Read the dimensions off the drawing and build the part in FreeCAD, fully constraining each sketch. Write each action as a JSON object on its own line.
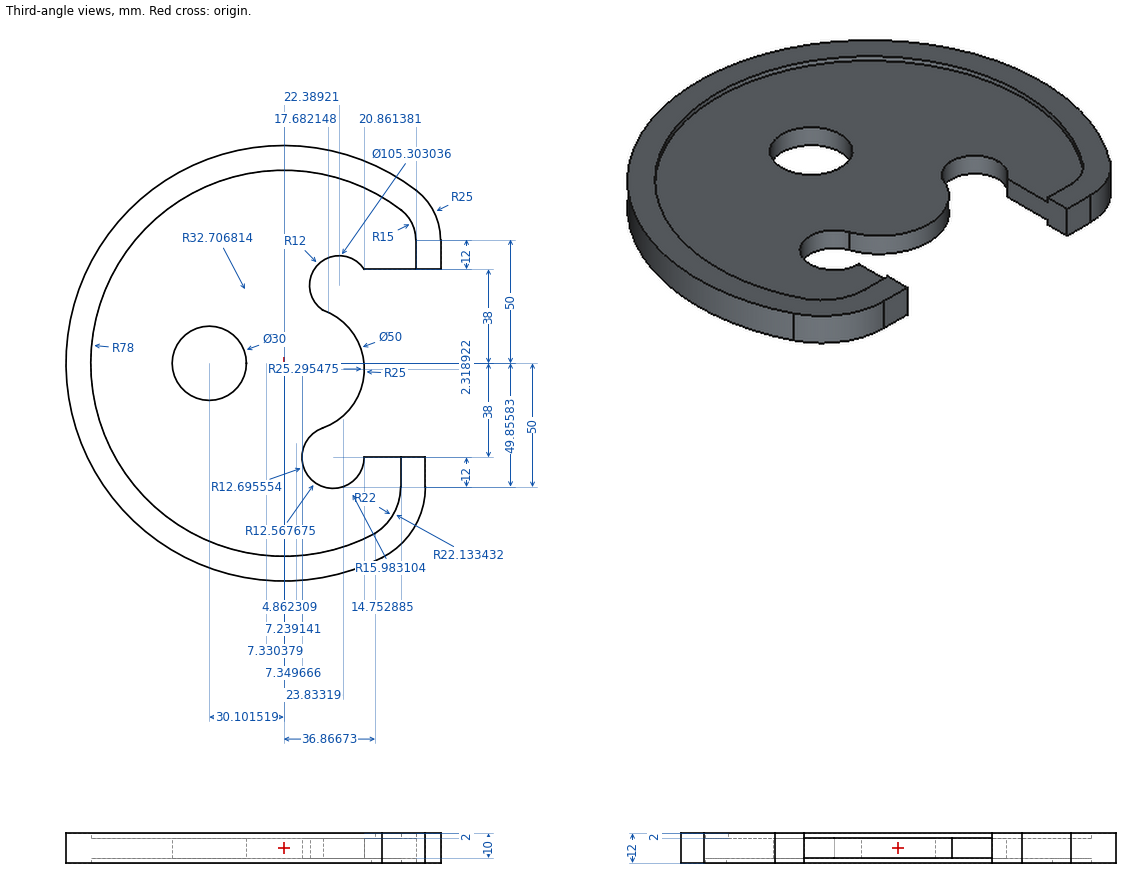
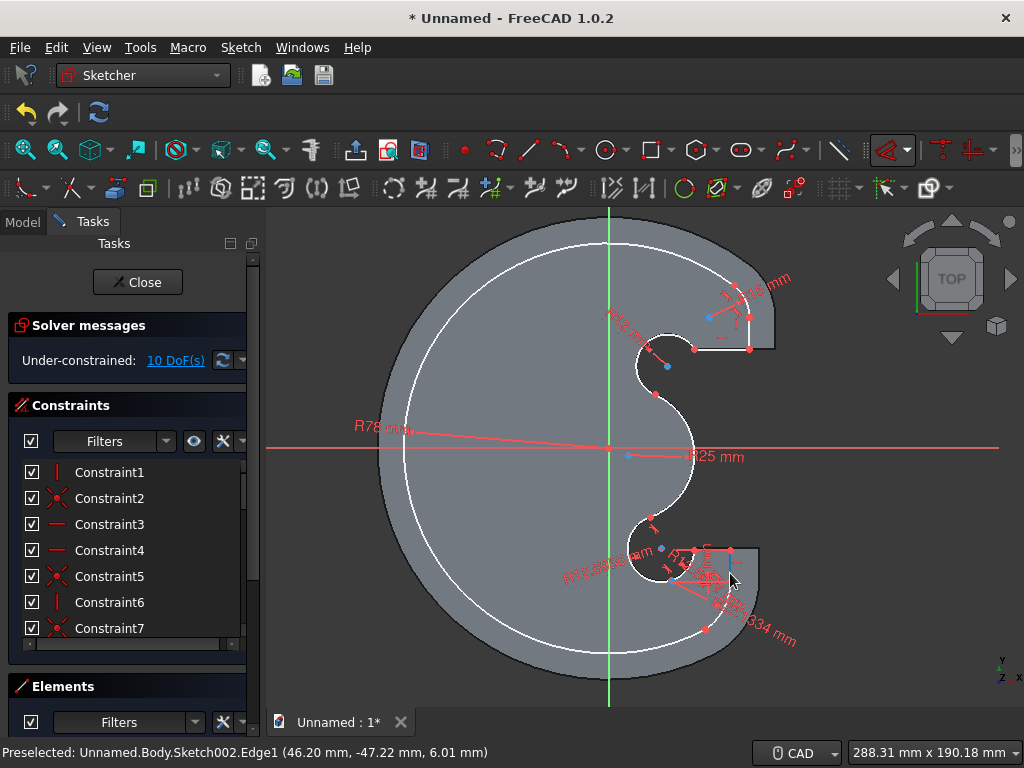
{"action": "scroll", "coordinate": [749, 340], "scroll_direction": "up", "scroll_amount": 2}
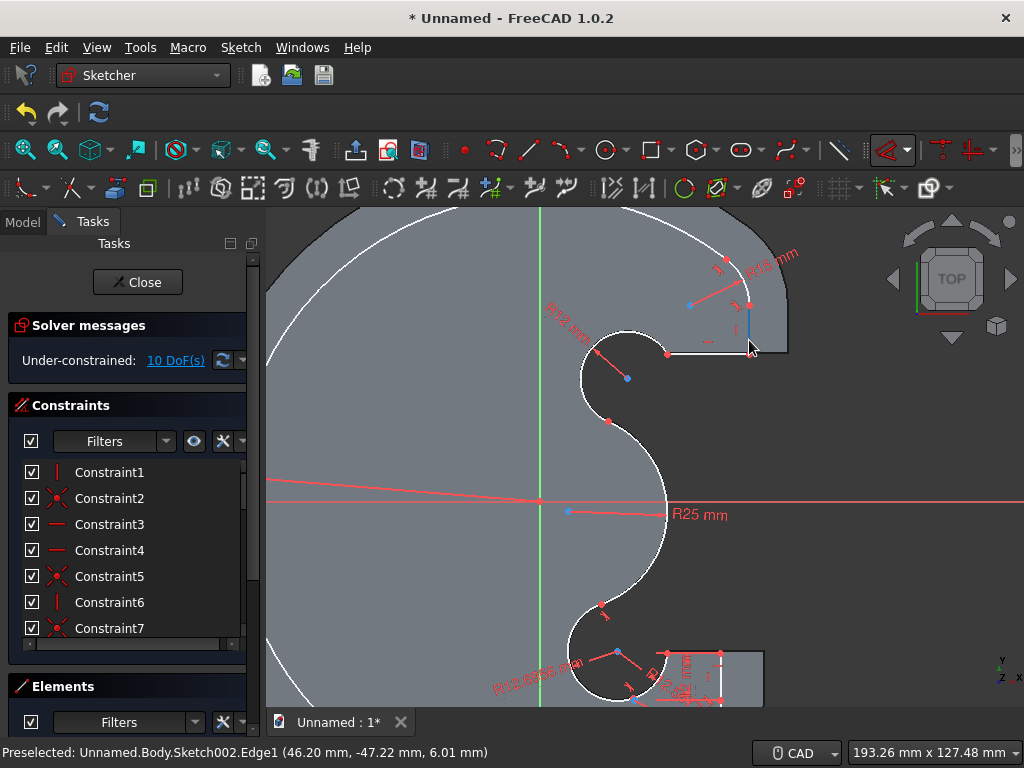
{"action": "left_click", "coordinate": [749, 340]}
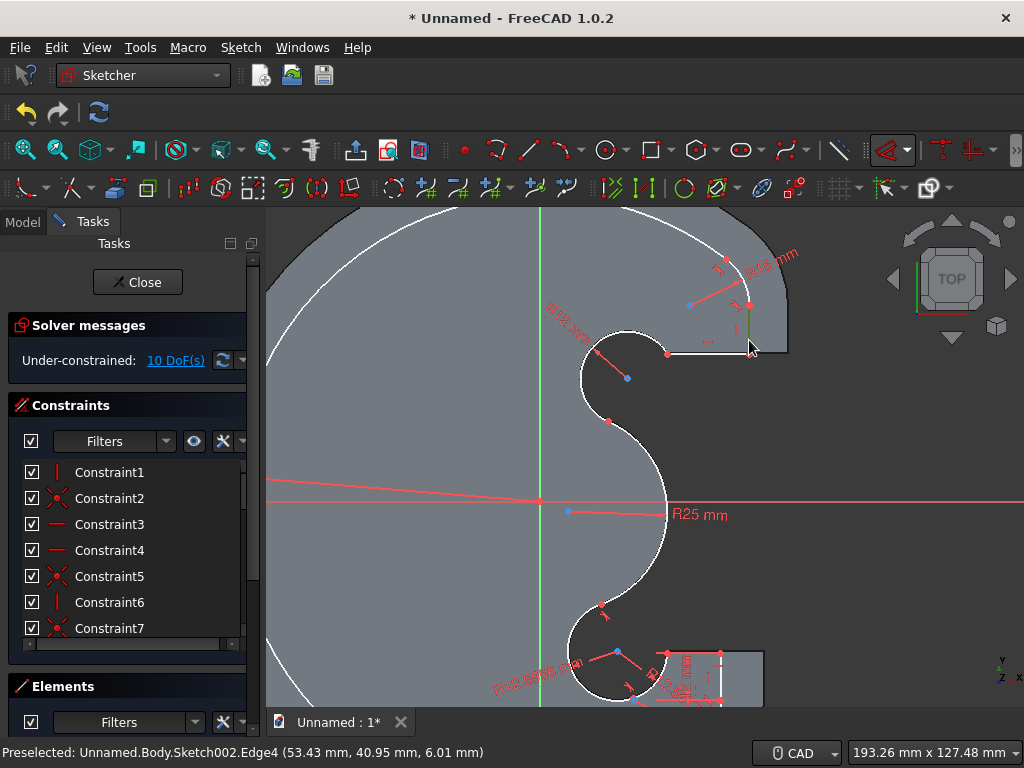
{"action": "key", "text": "i"}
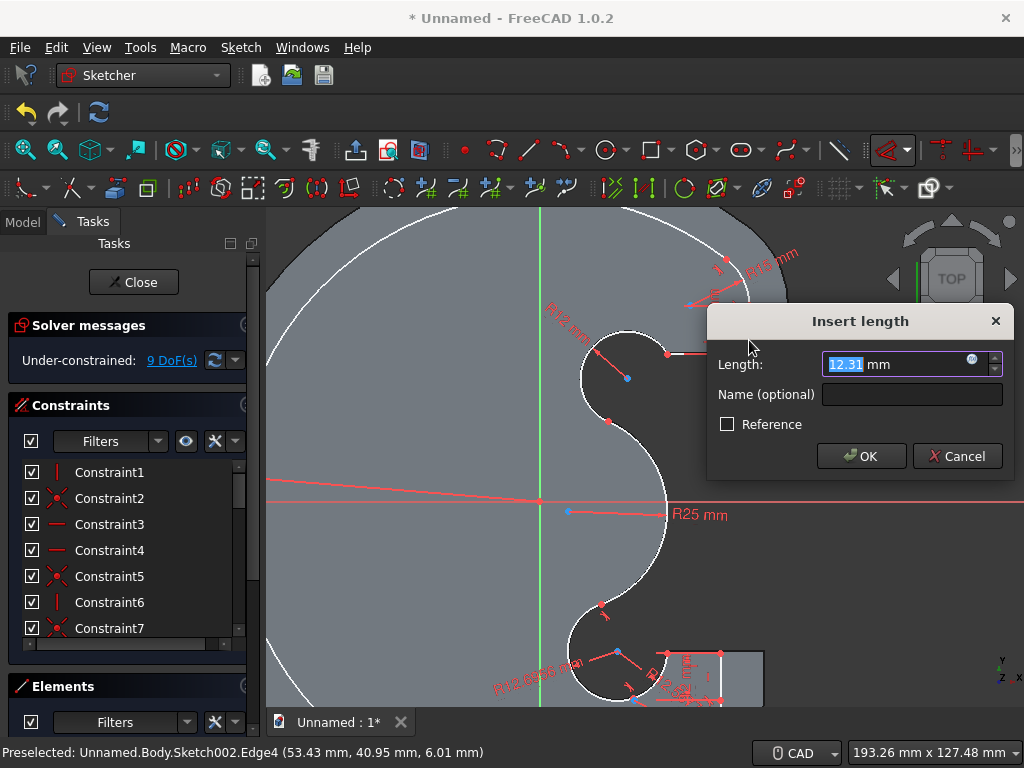
{"action": "type", "text": "12"}
{"action": "key", "text": "Return"}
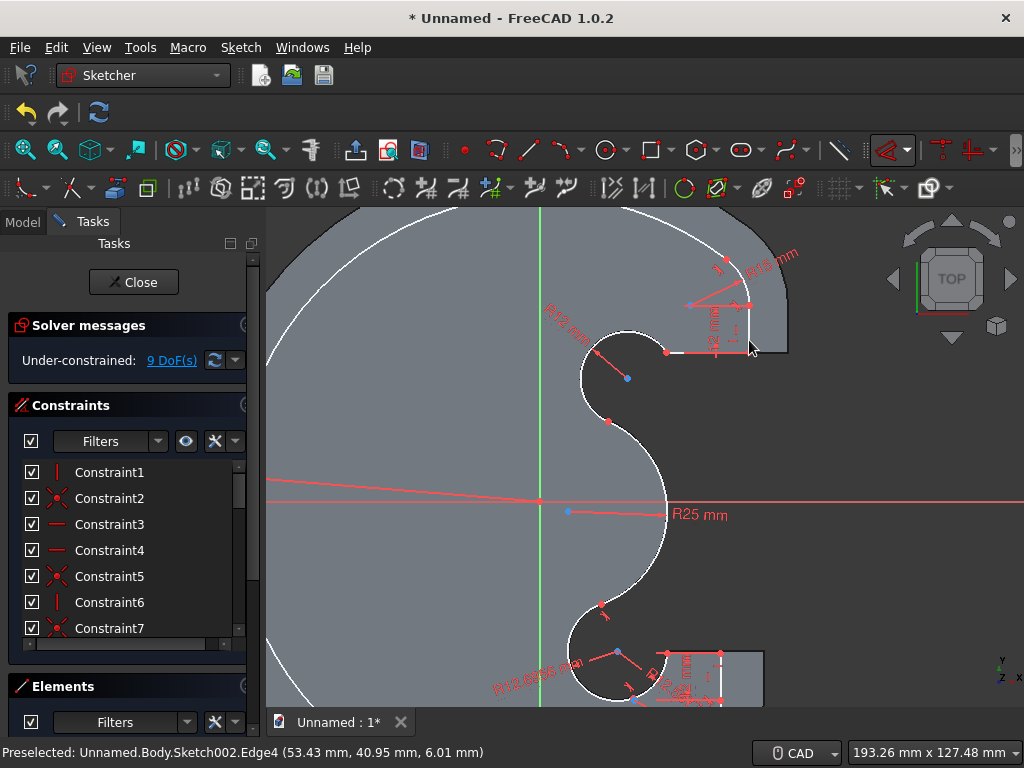
{"action": "scroll", "coordinate": [749, 339], "scroll_direction": "down", "scroll_amount": 2}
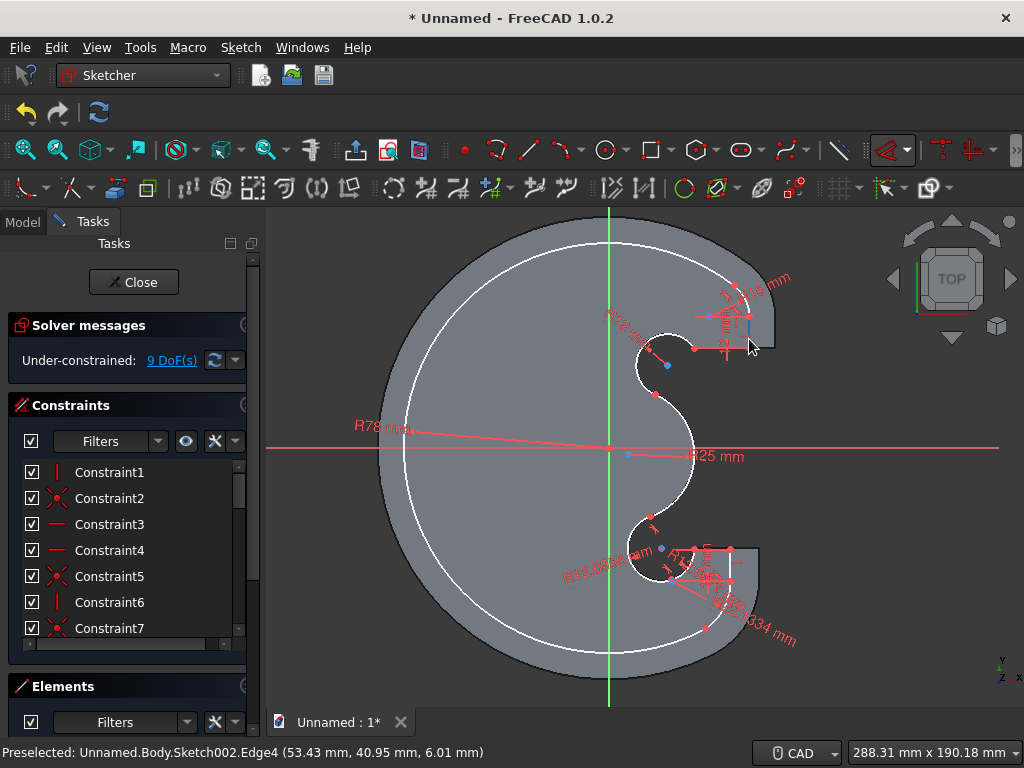
{"action": "left_click", "coordinate": [730, 581]}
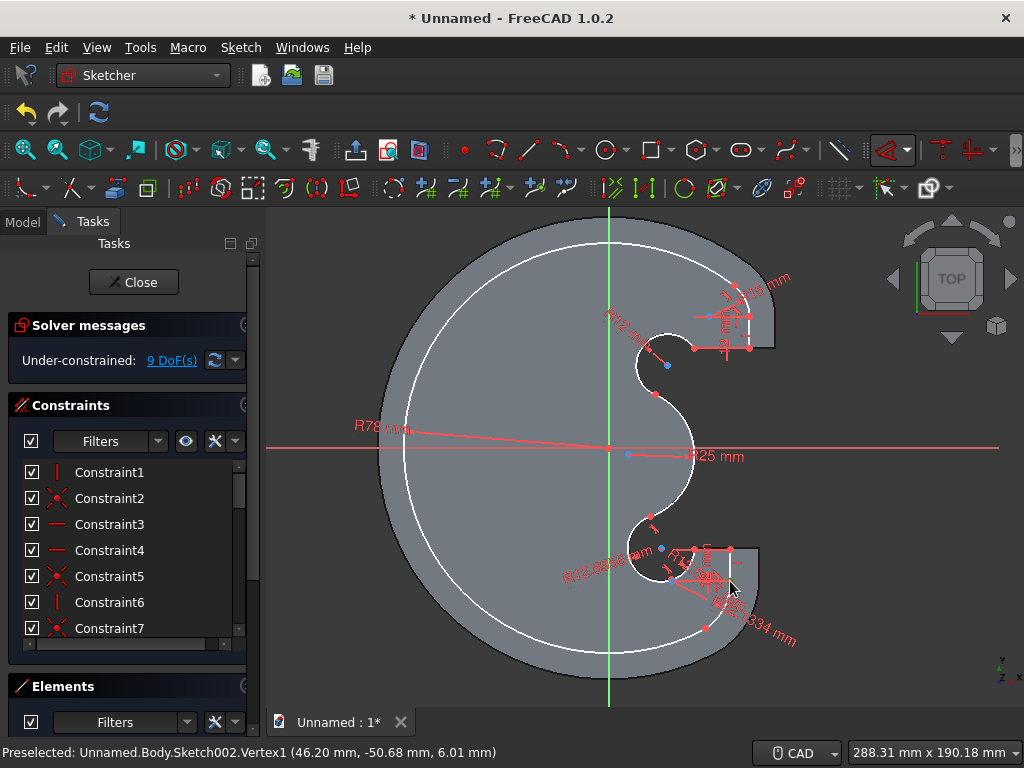
{"action": "key", "text": "i"}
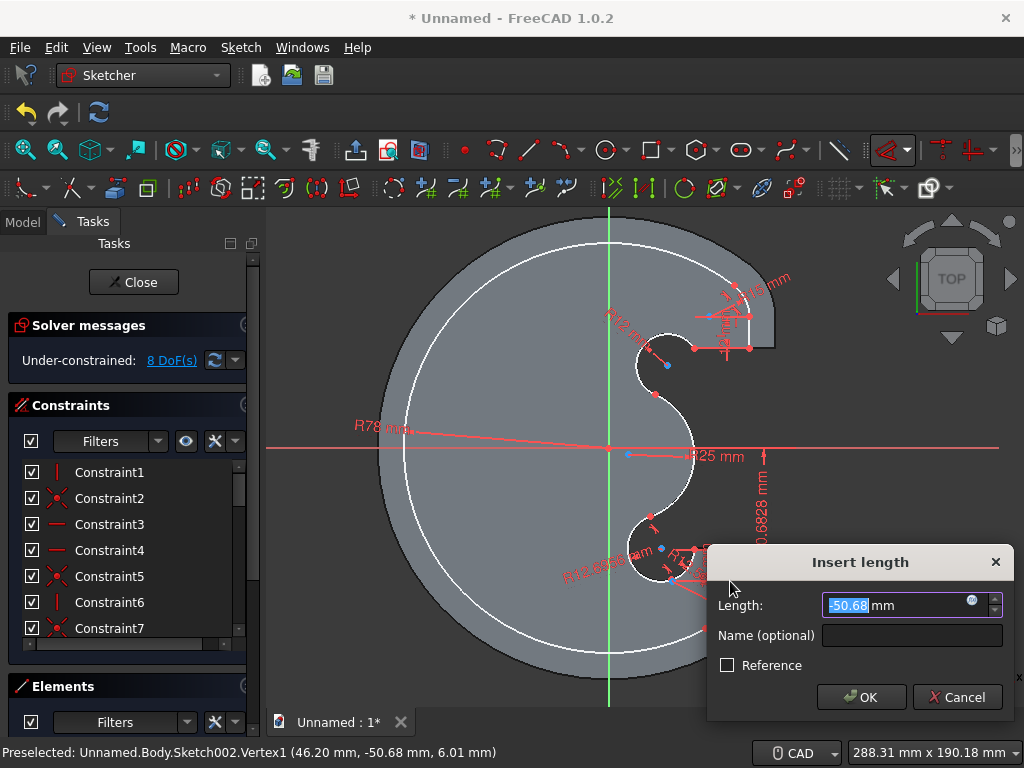
{"action": "type", "text": "-50"}
{"action": "key", "text": "Return"}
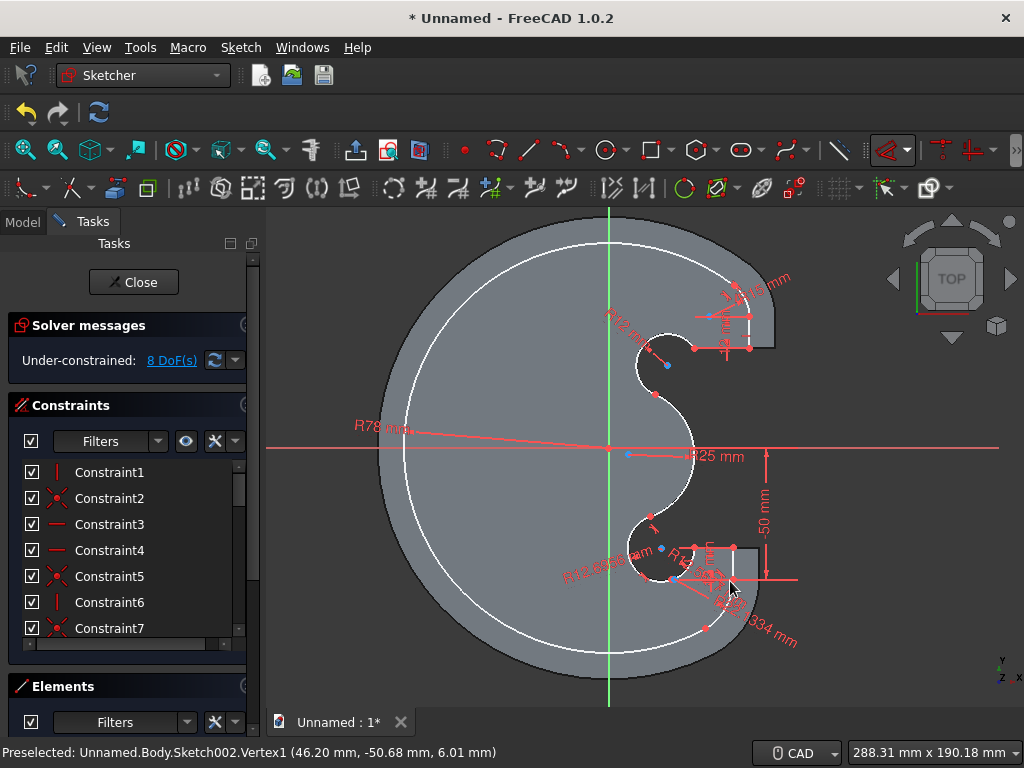
{"action": "left_click", "coordinate": [694, 348]}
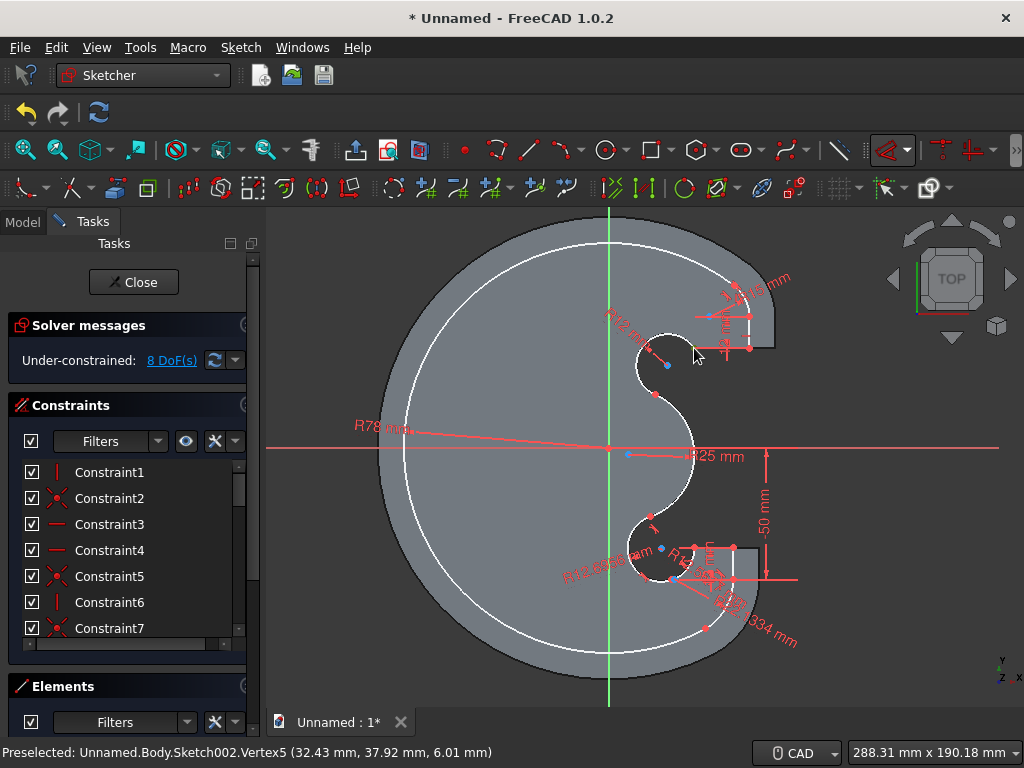
{"action": "key", "text": "i"}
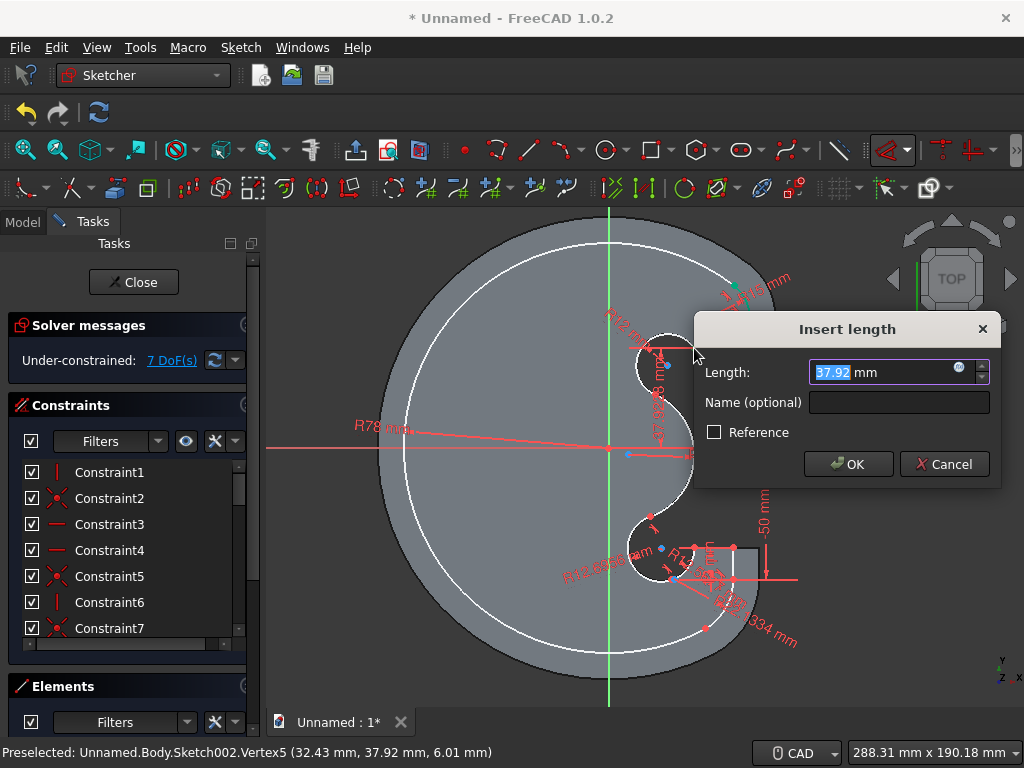
{"action": "type", "text": "38"}
{"action": "key", "text": "Return"}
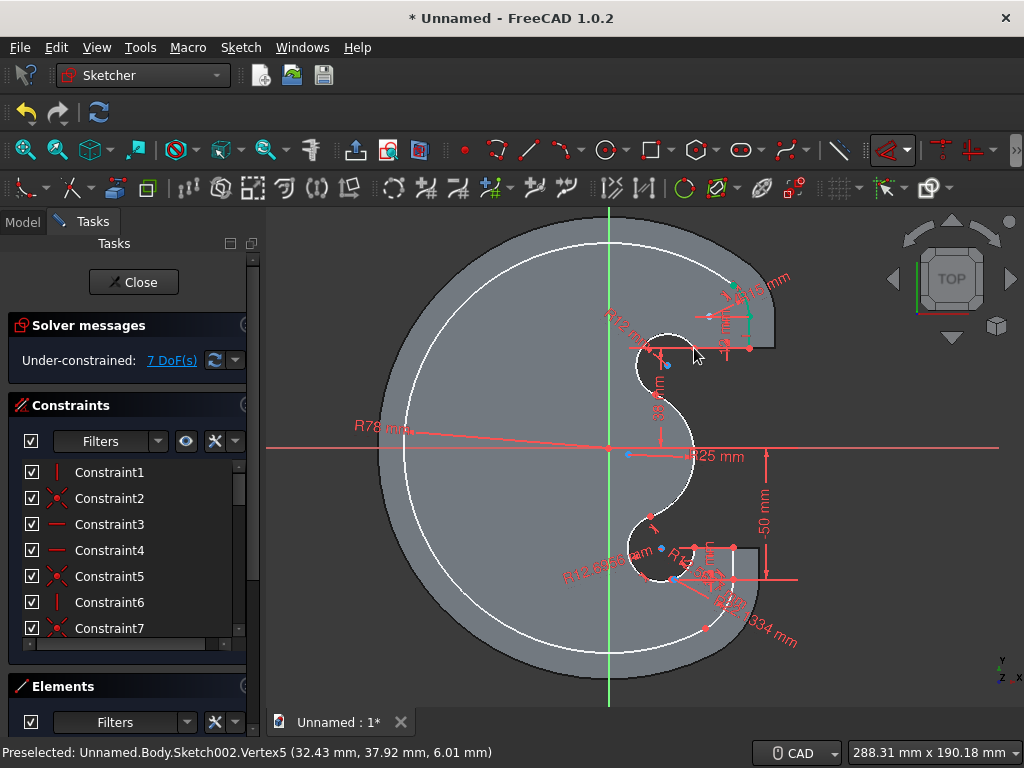
{"action": "scroll", "coordinate": [661, 549], "scroll_direction": "up", "scroll_amount": 13}